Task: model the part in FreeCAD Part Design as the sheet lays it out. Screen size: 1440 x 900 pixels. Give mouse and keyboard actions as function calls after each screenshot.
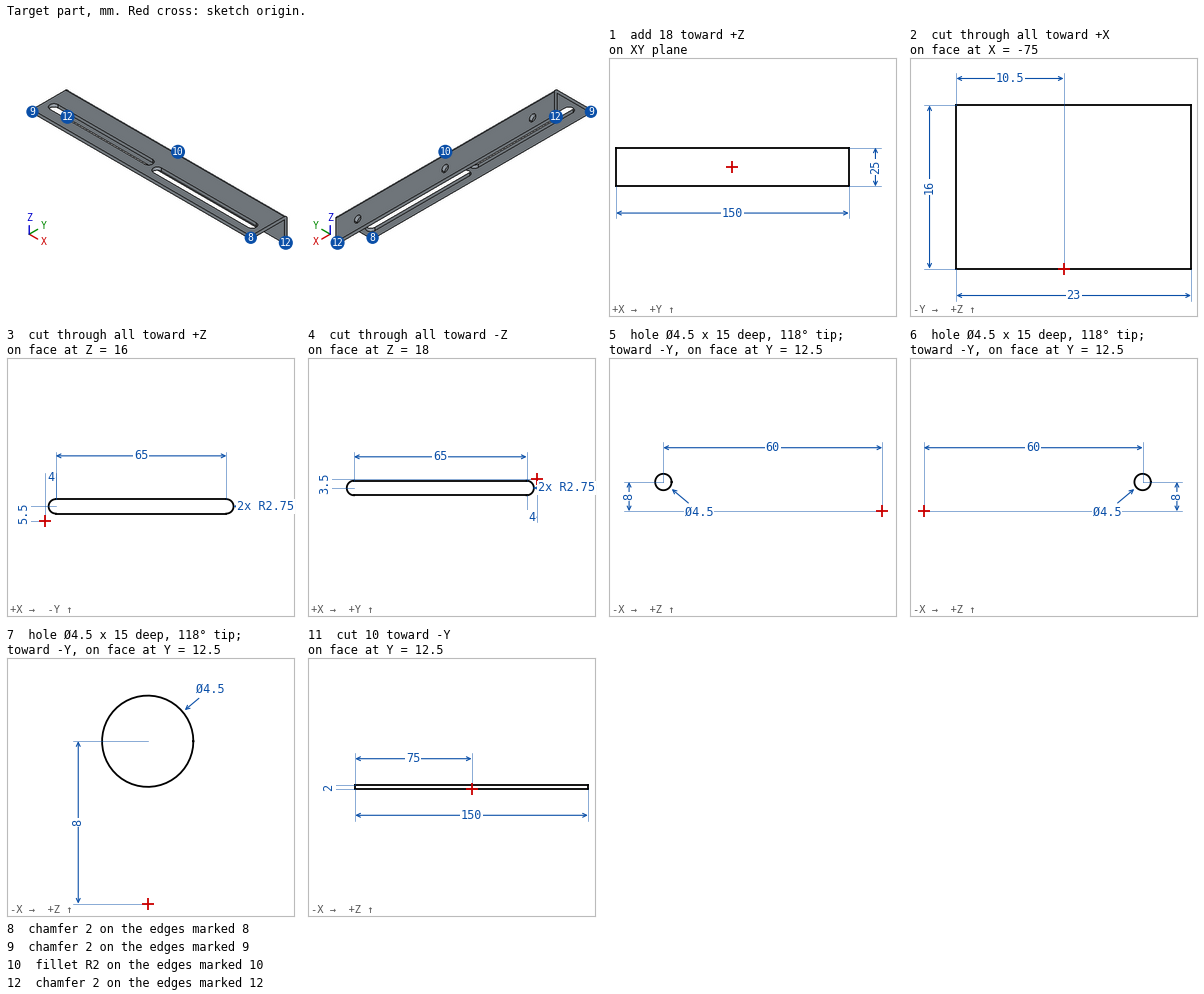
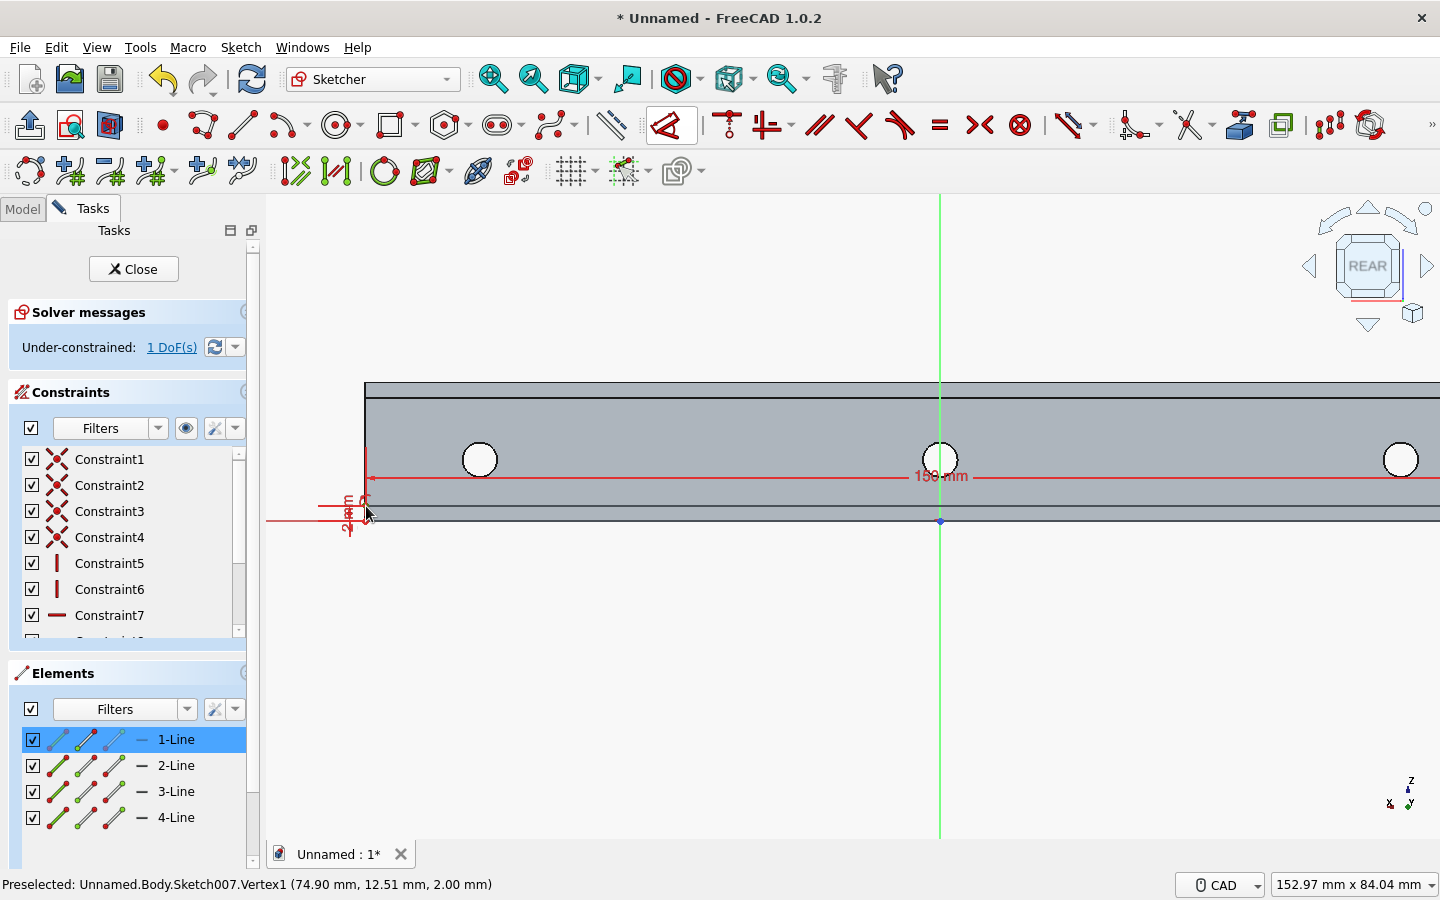
click(692, 126)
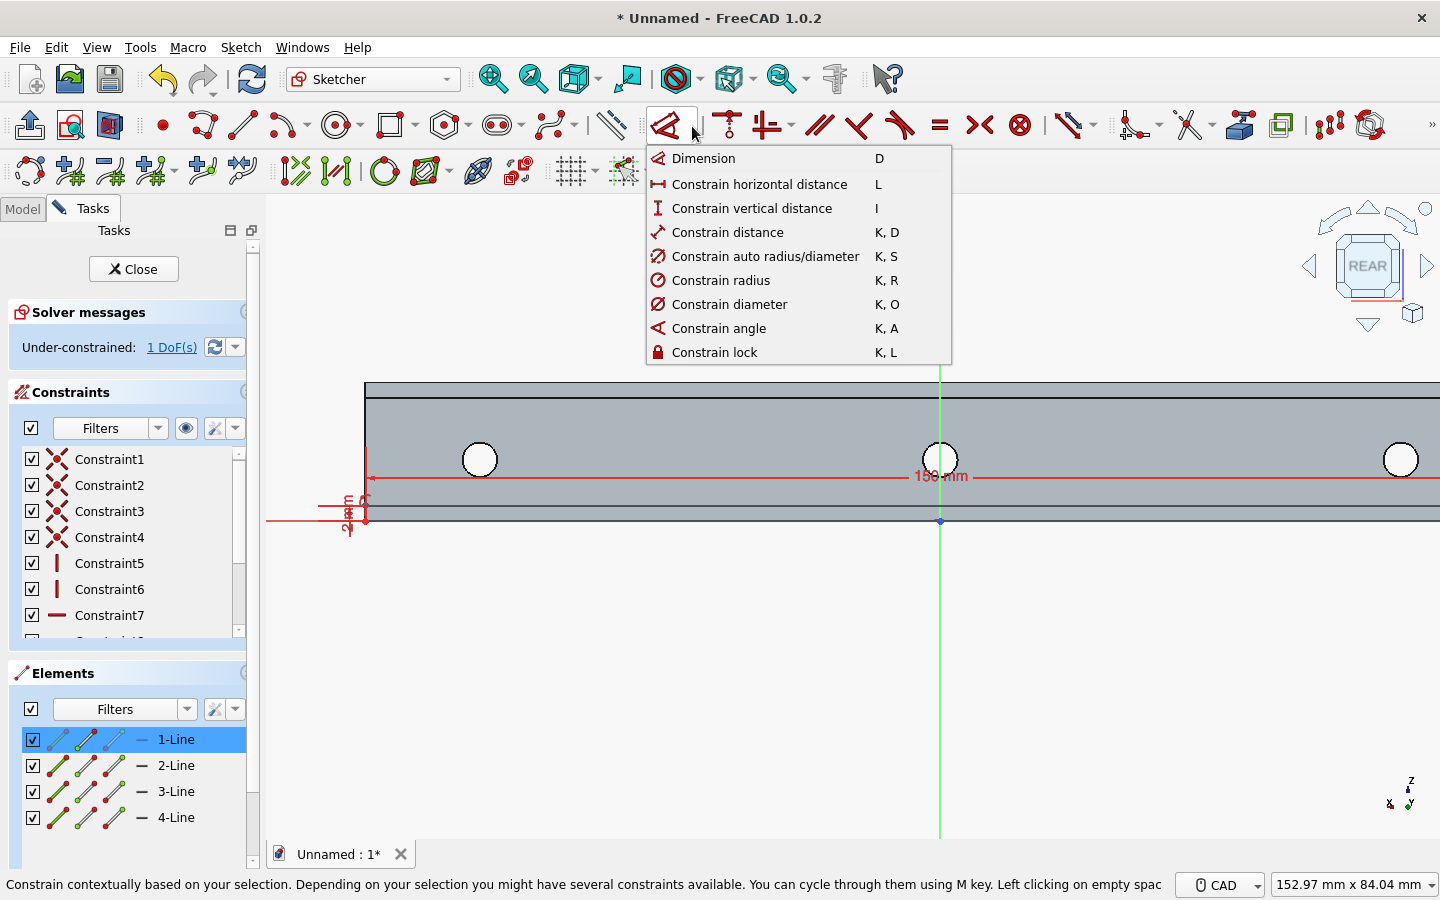
click(799, 184)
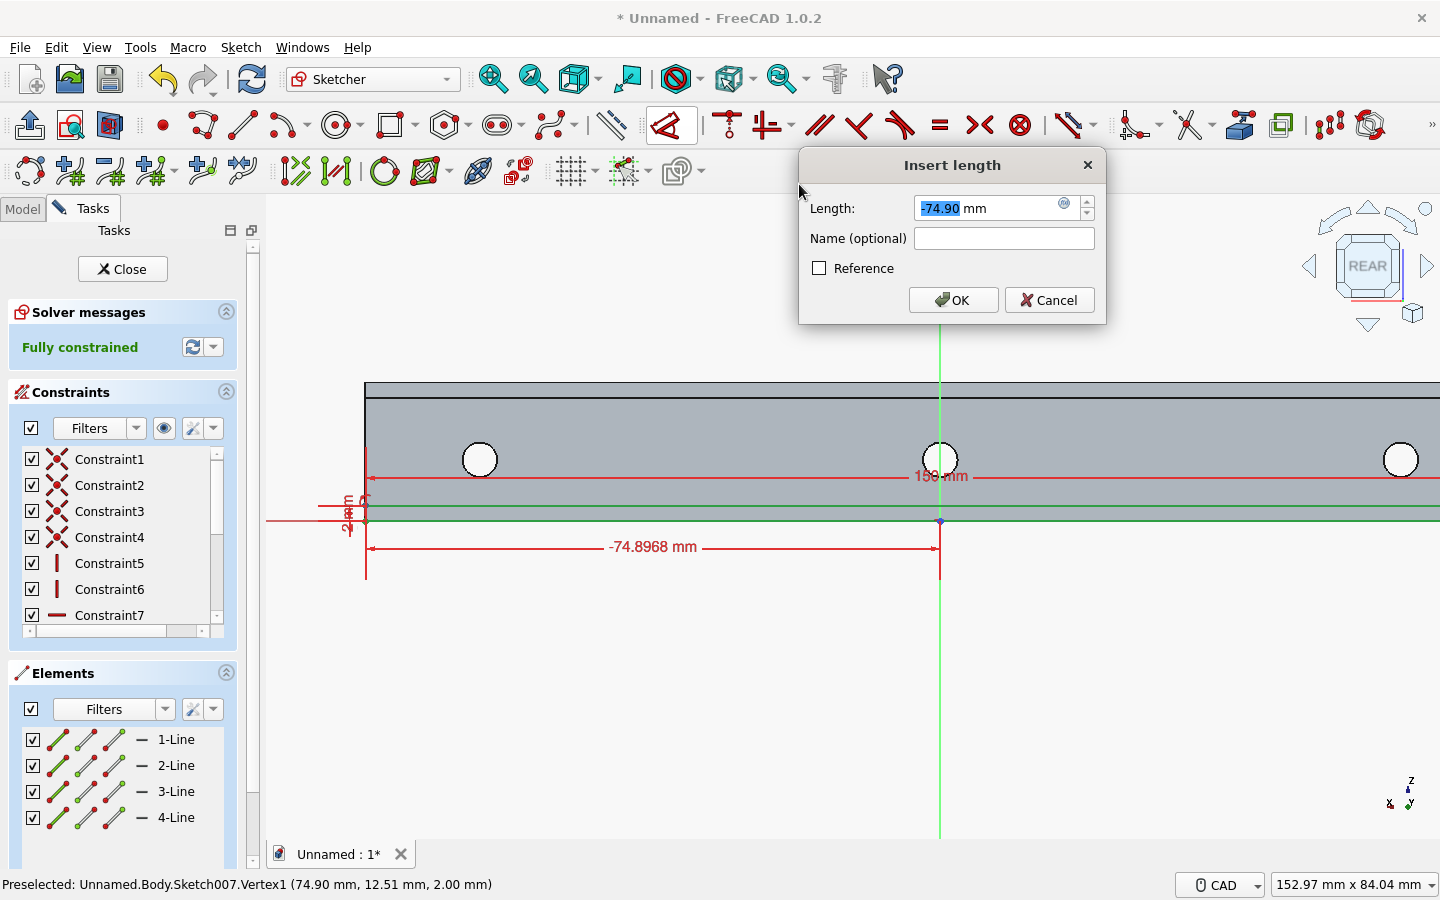
text(-75)
key(Return)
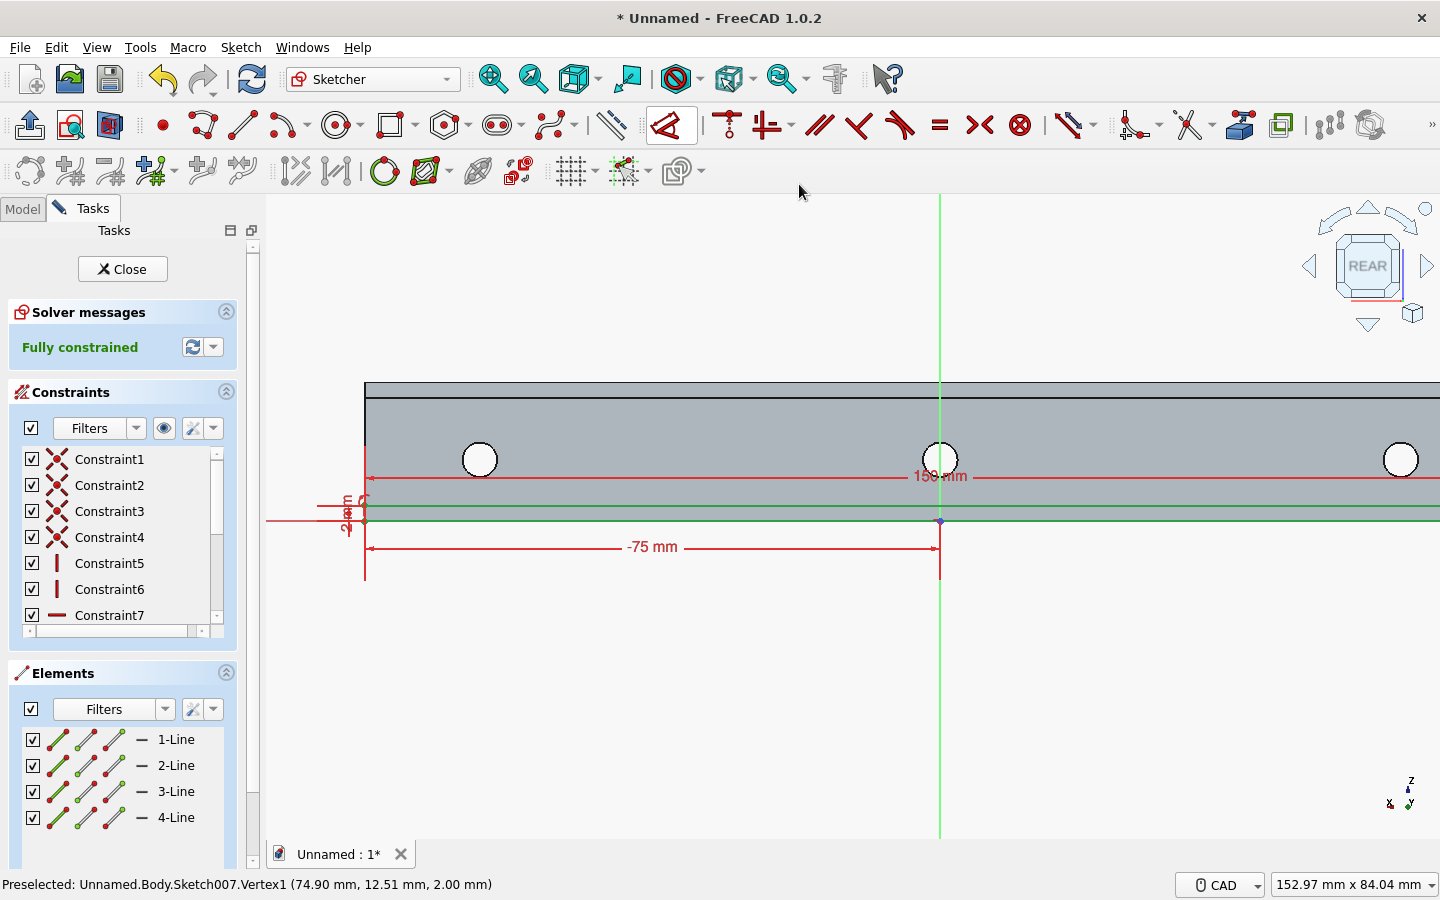
click(123, 269)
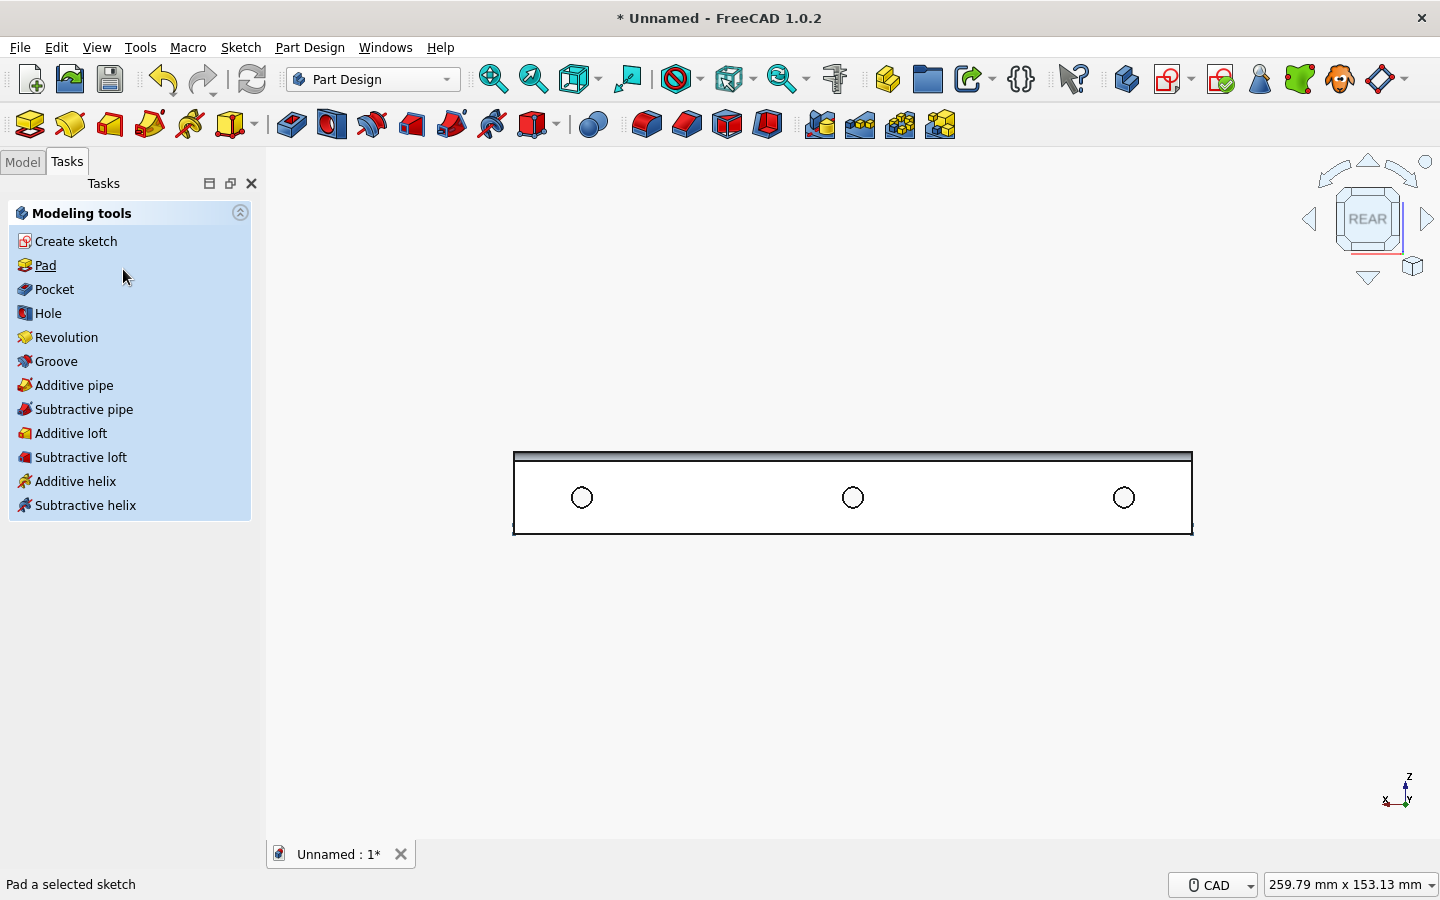
click(292, 124)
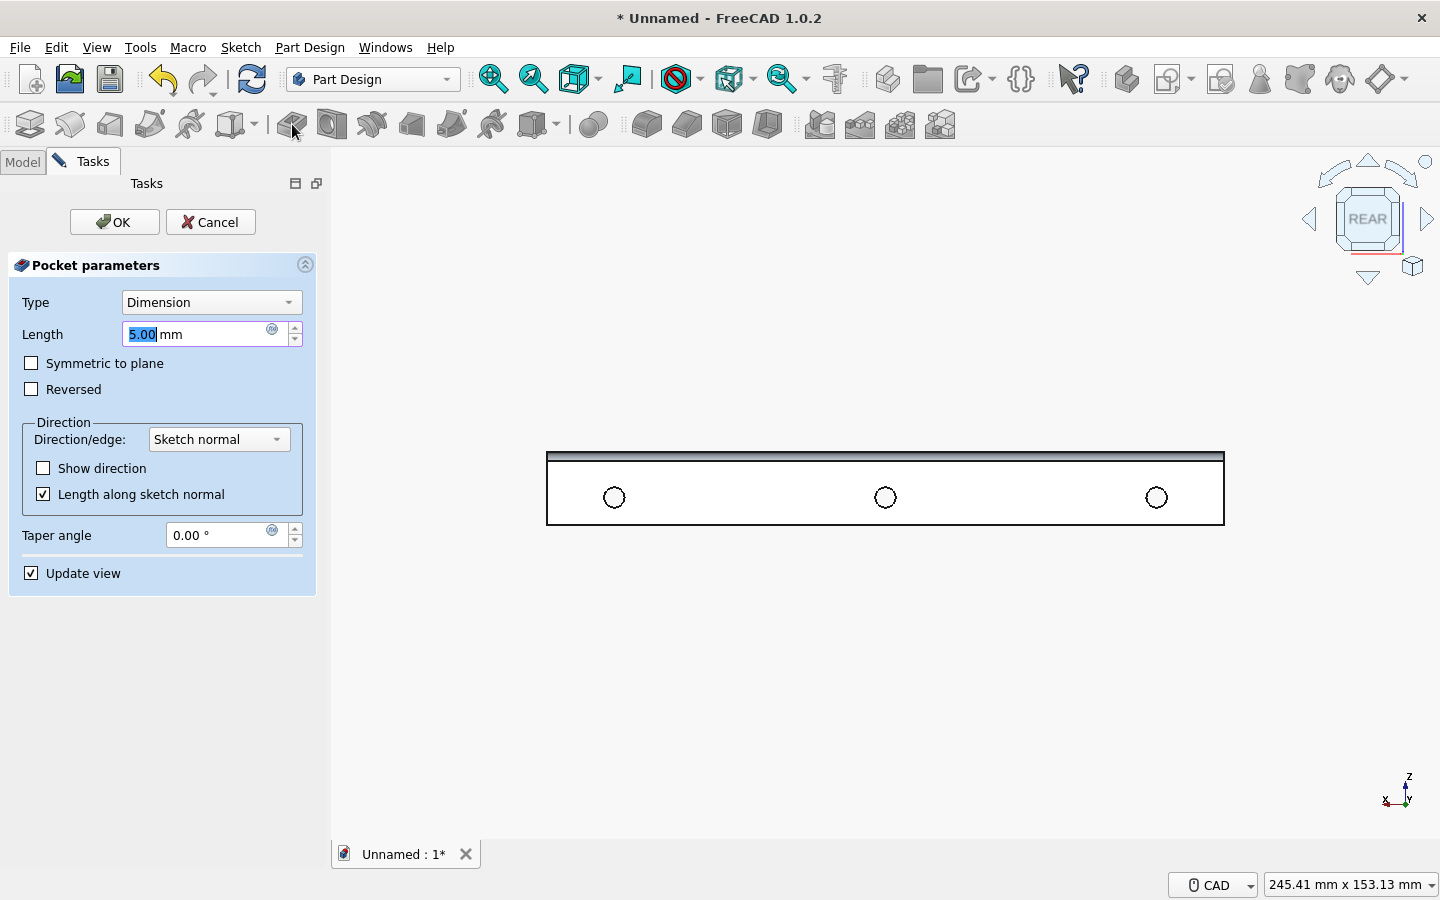
text(10)
key(Tab)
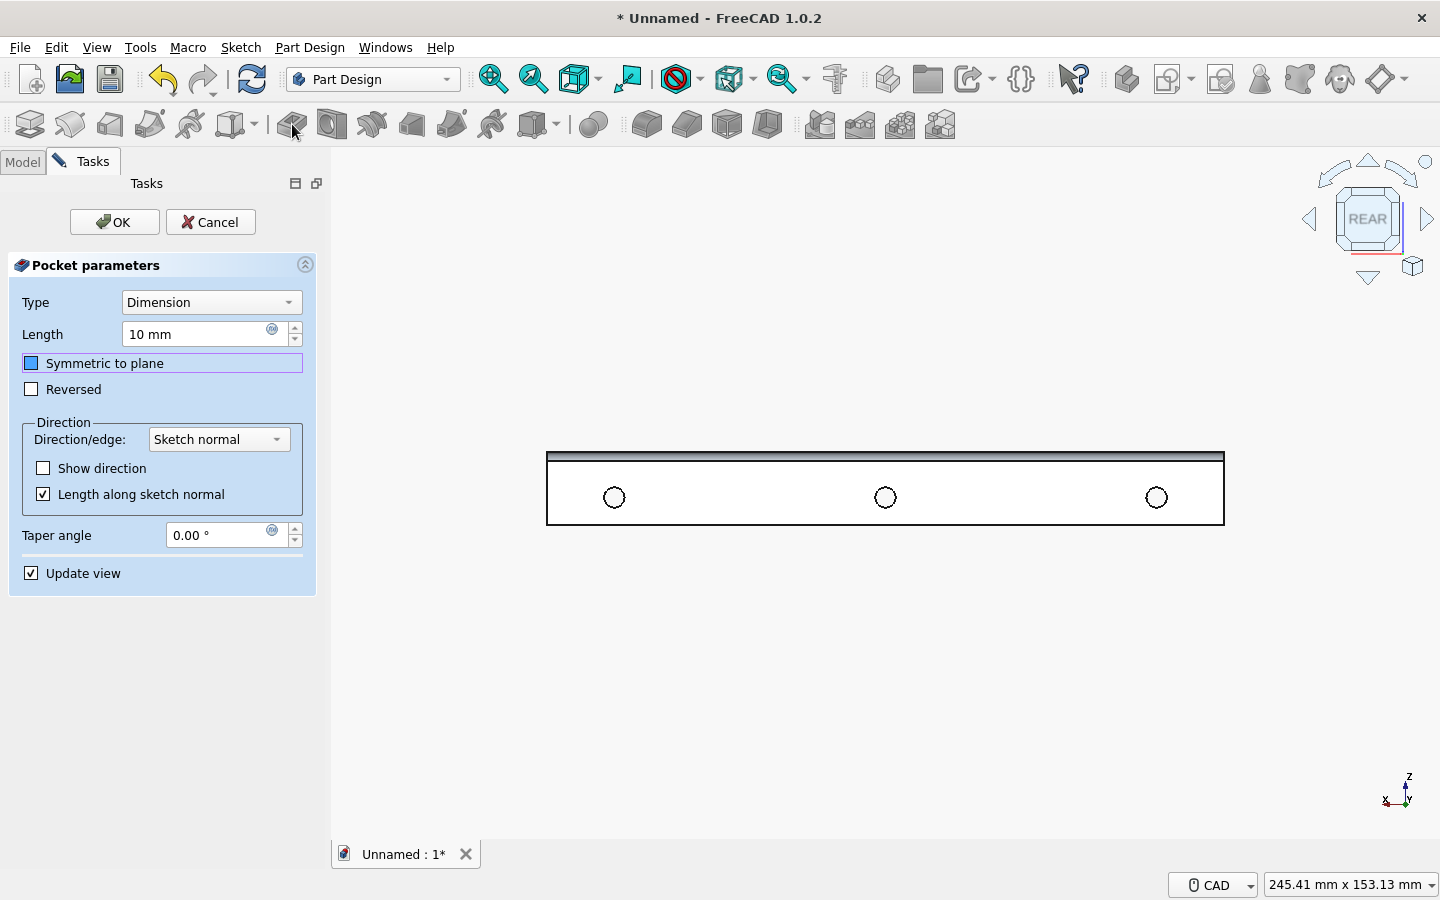
click(115, 222)